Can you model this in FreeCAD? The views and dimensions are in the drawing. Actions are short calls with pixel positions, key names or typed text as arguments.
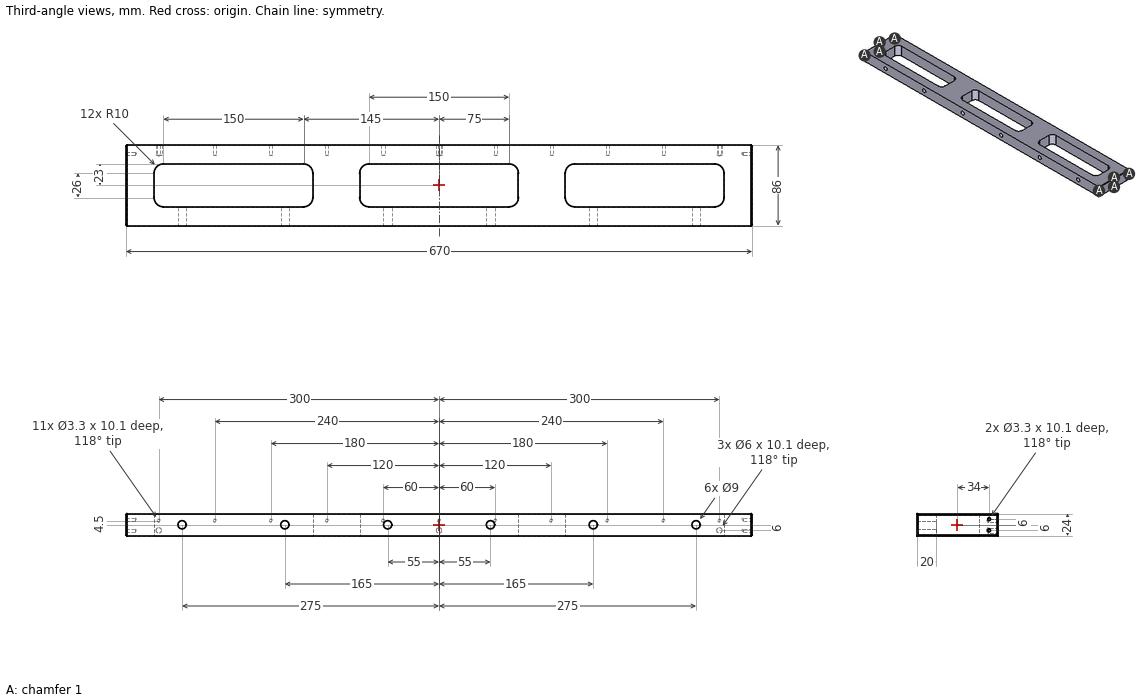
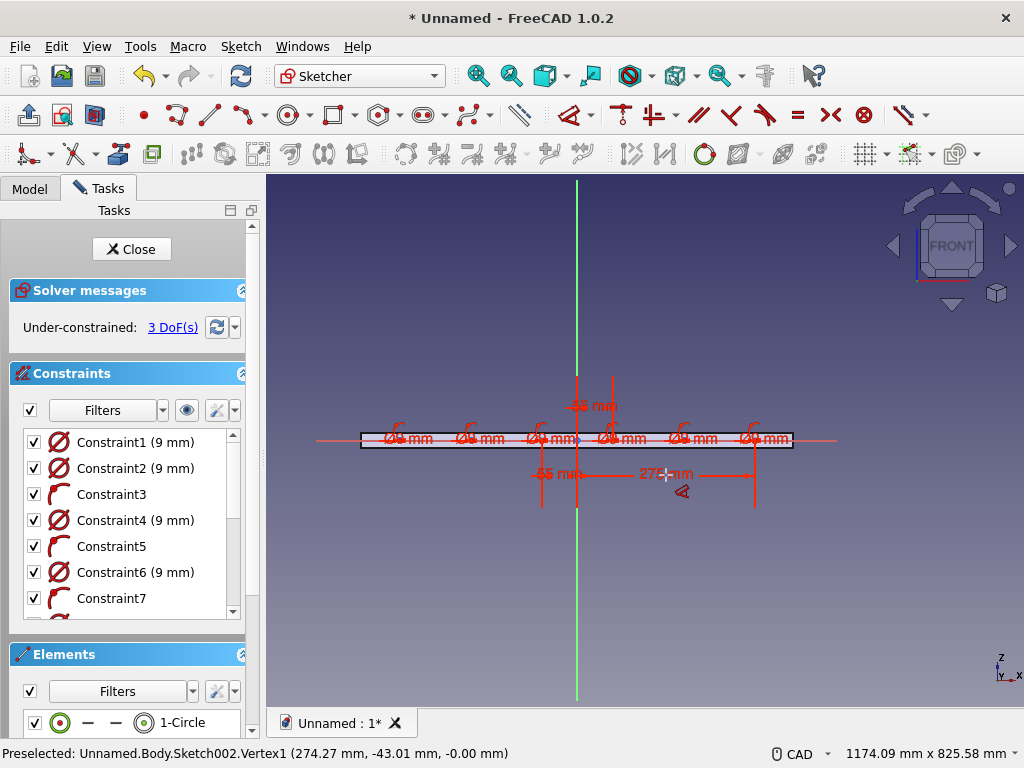
click(399, 441)
click(488, 475)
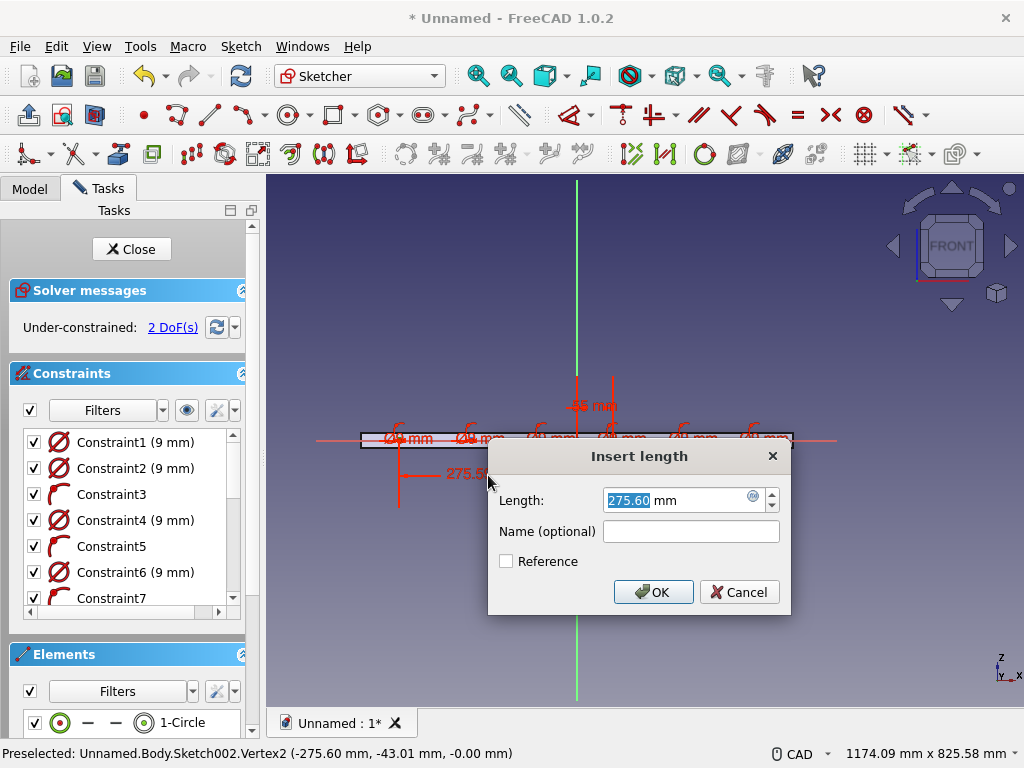
text(275)
key(Return)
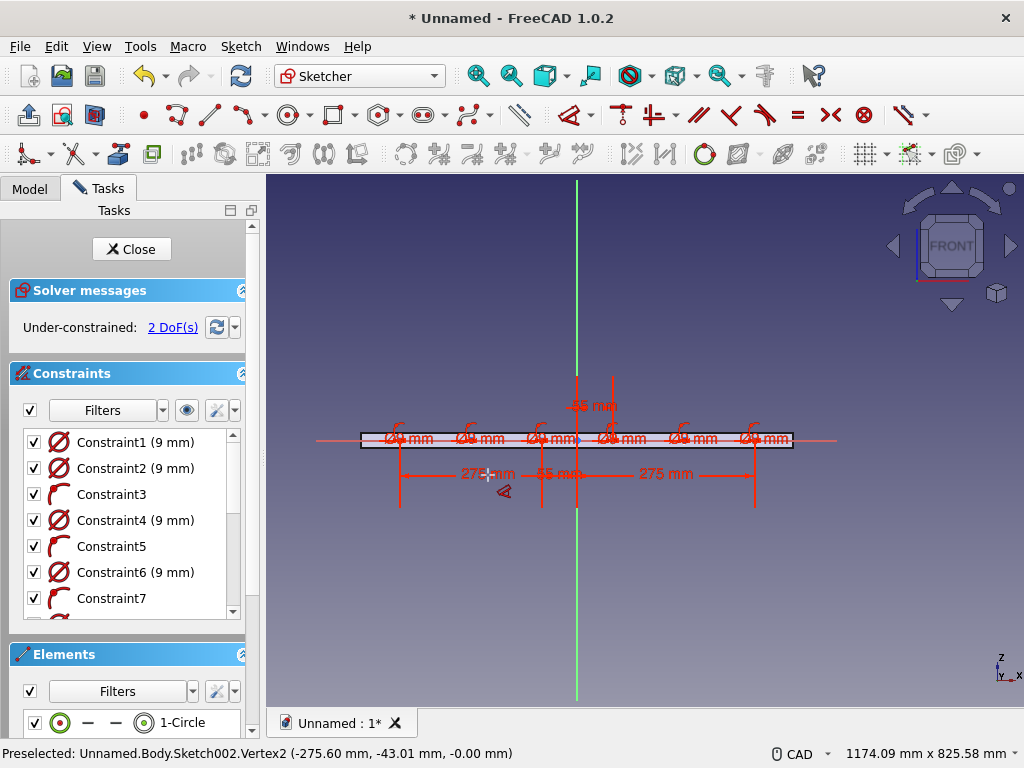
click(471, 441)
click(524, 407)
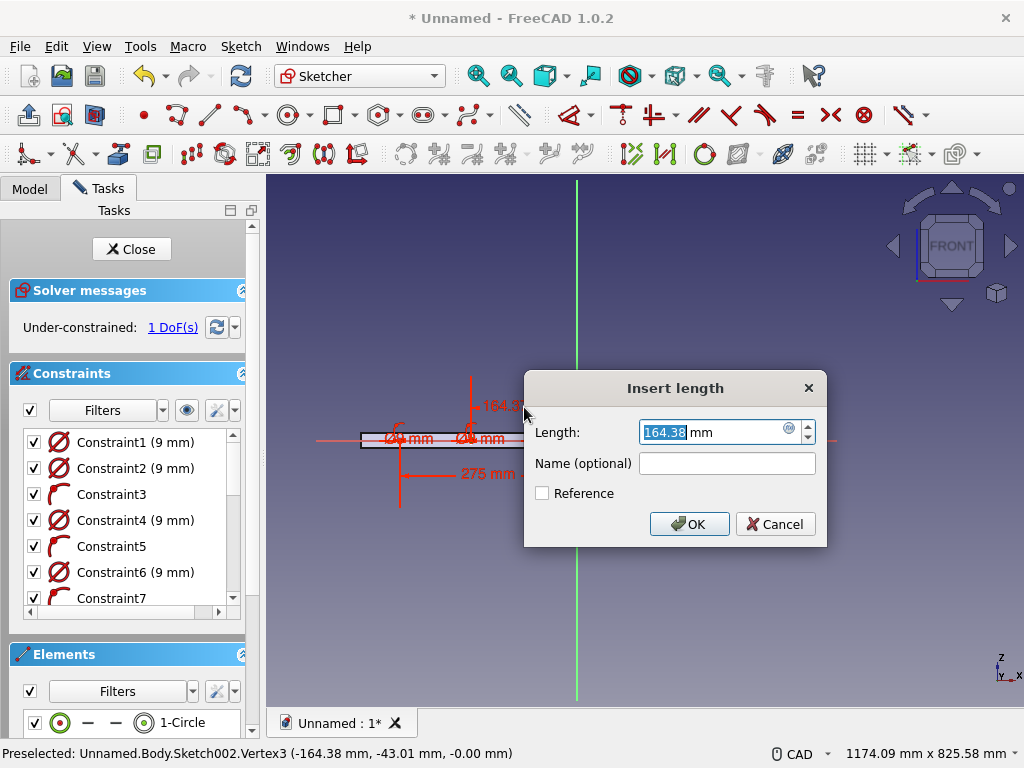
text(165)
key(Return)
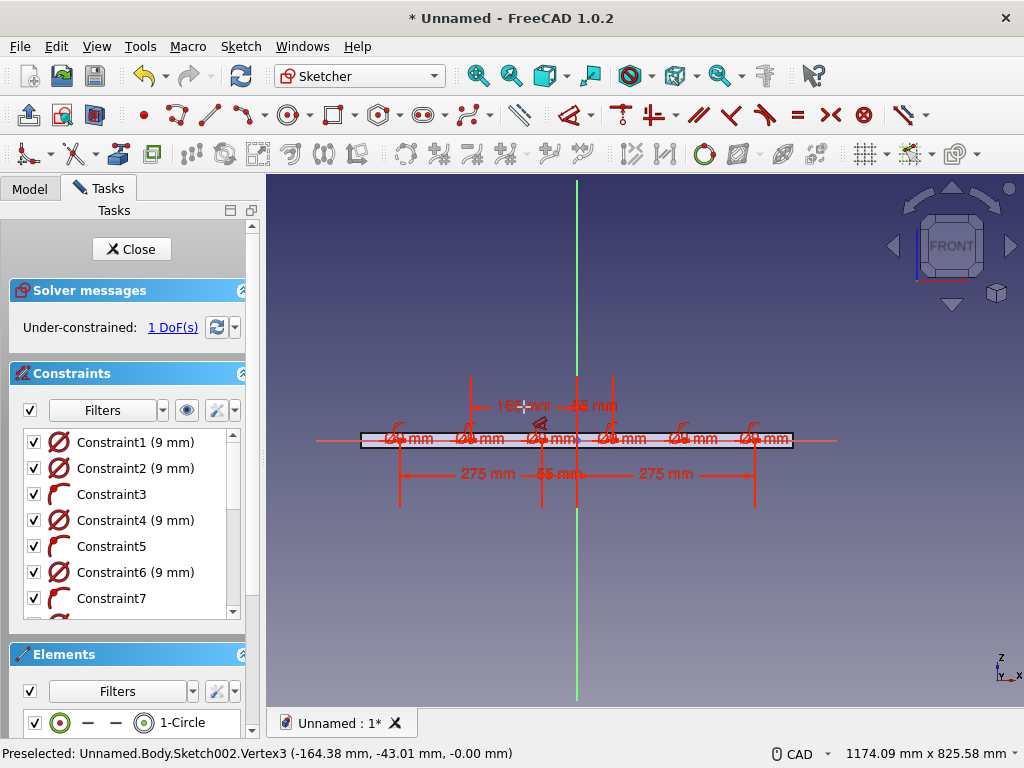
click(684, 441)
click(668, 407)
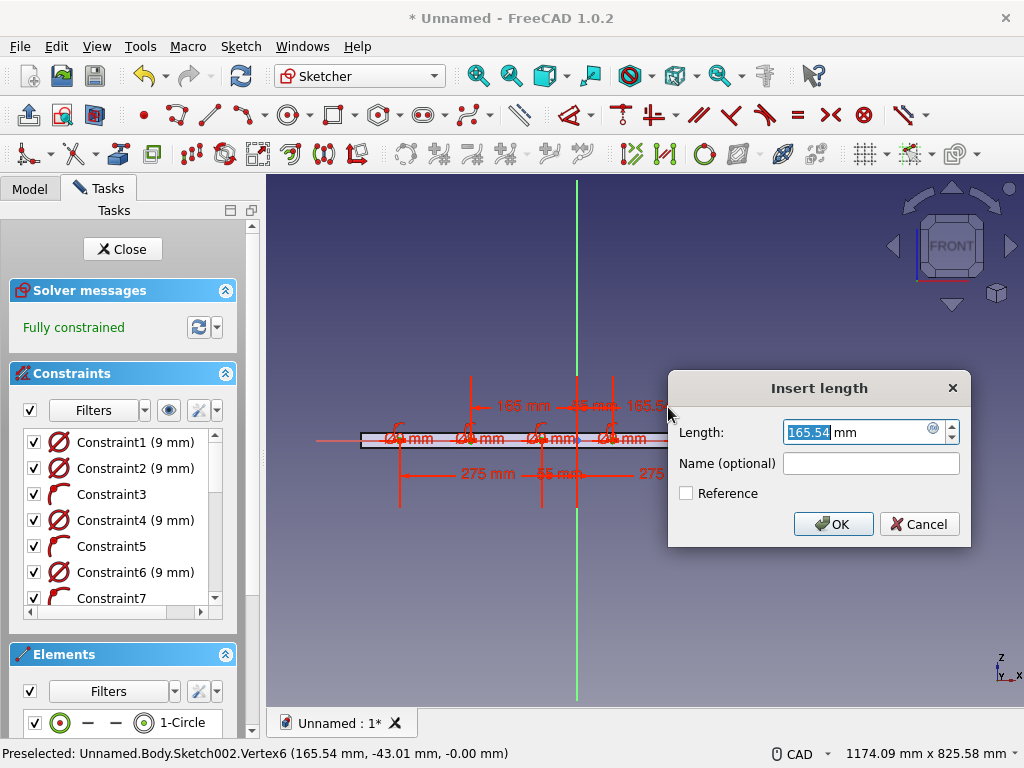
text(165)
key(Return)
key(Escape)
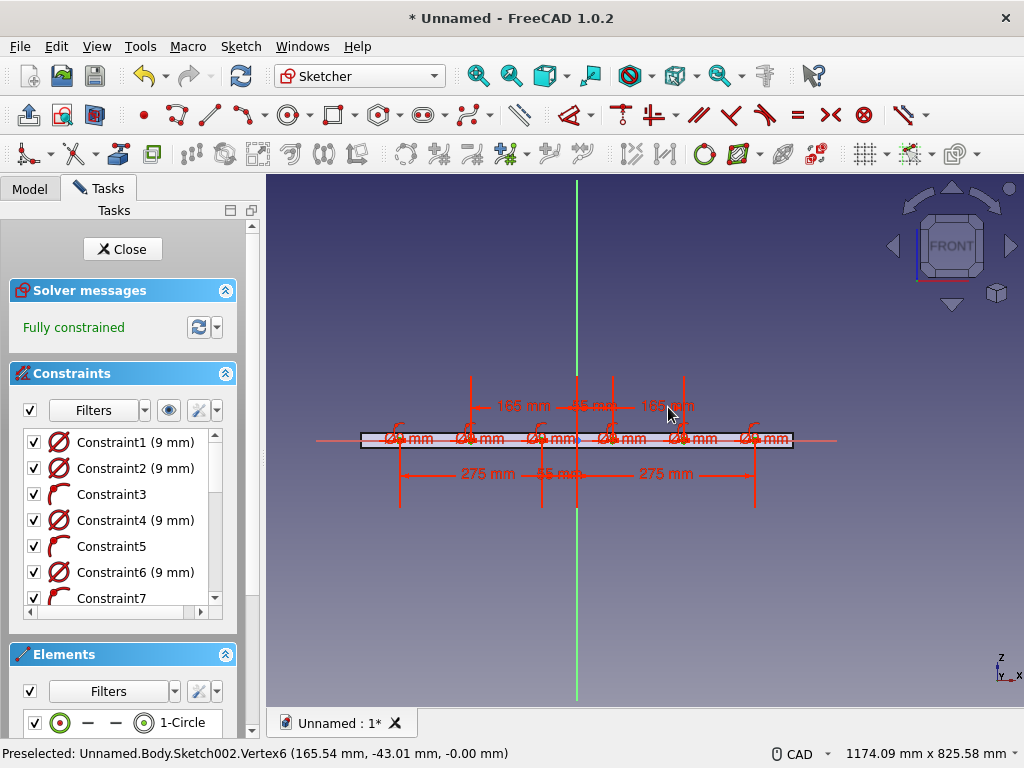
click(123, 249)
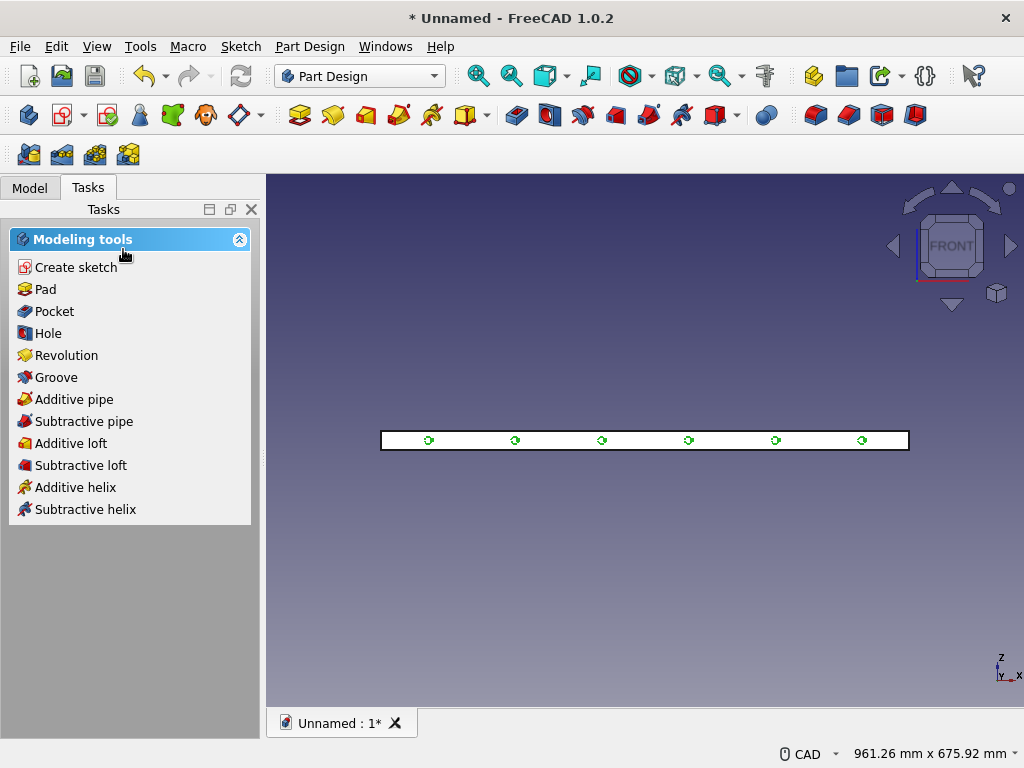
click(517, 116)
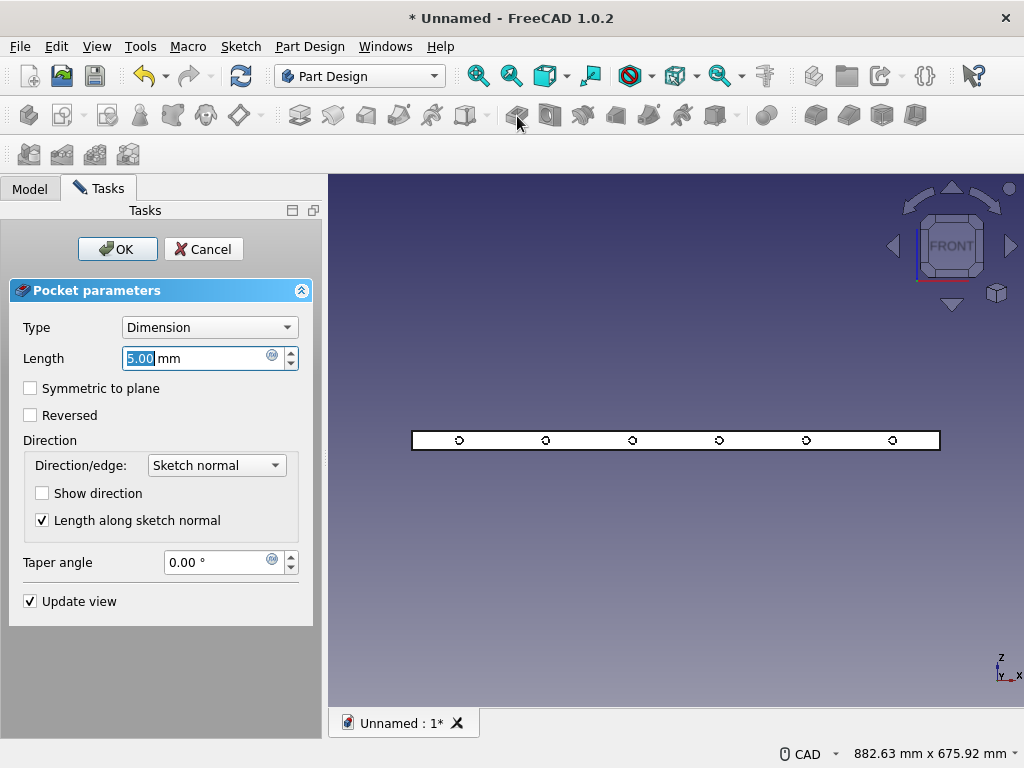
text(20)
key(Tab)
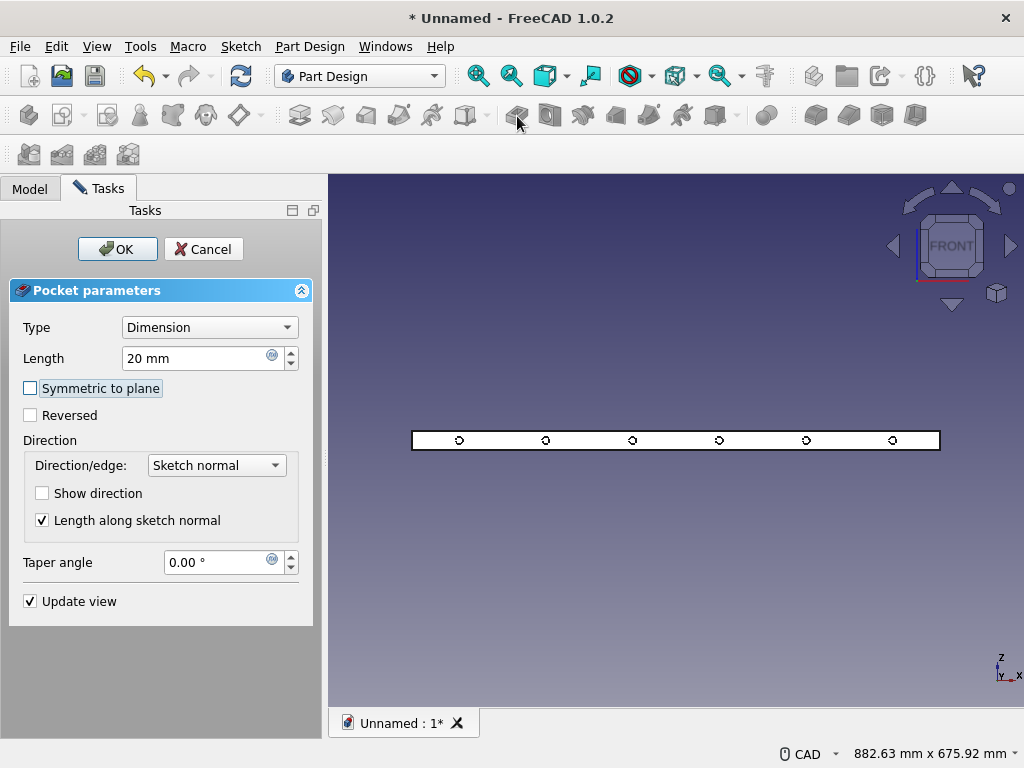
click(118, 249)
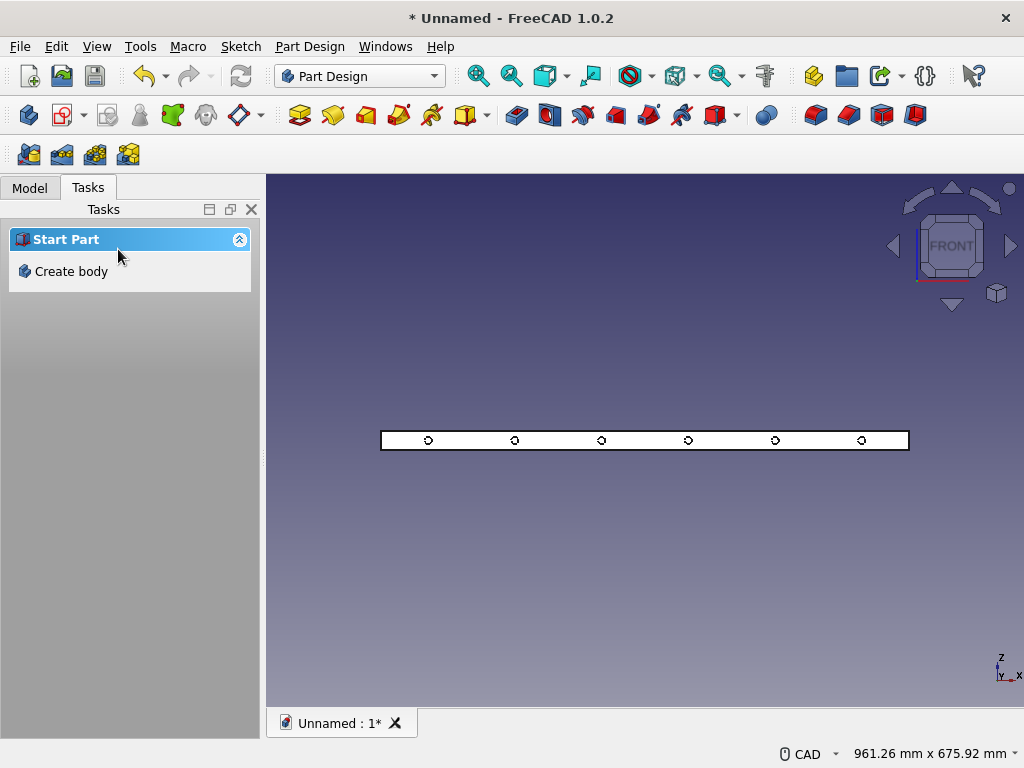
key(4)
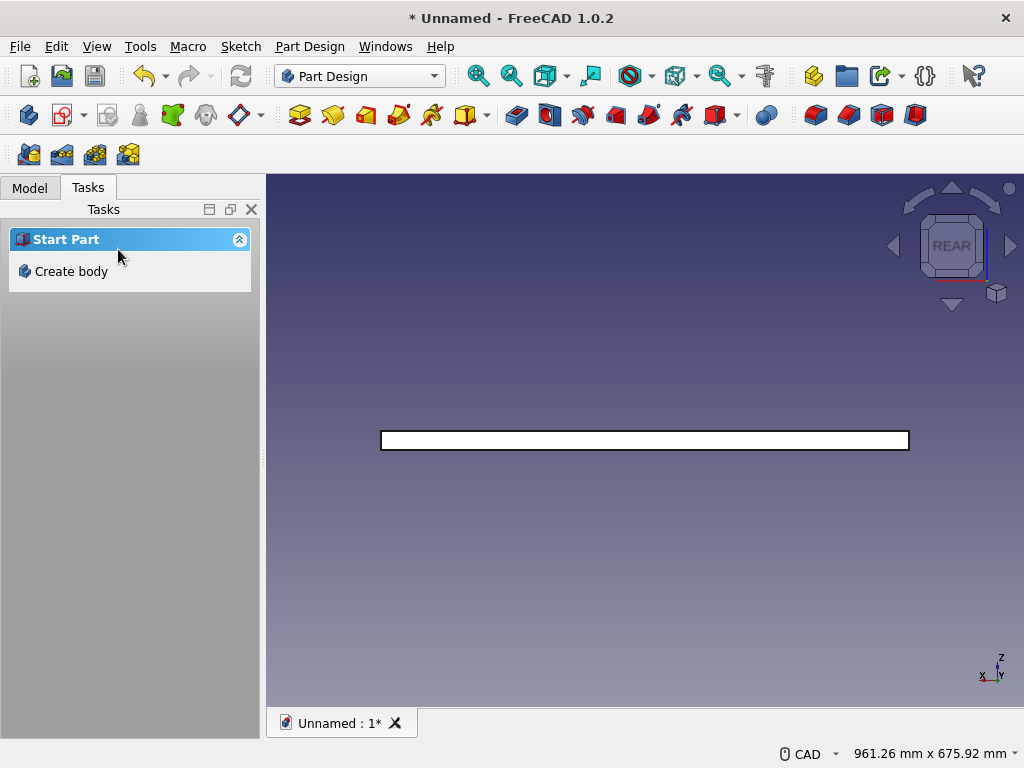
click(419, 439)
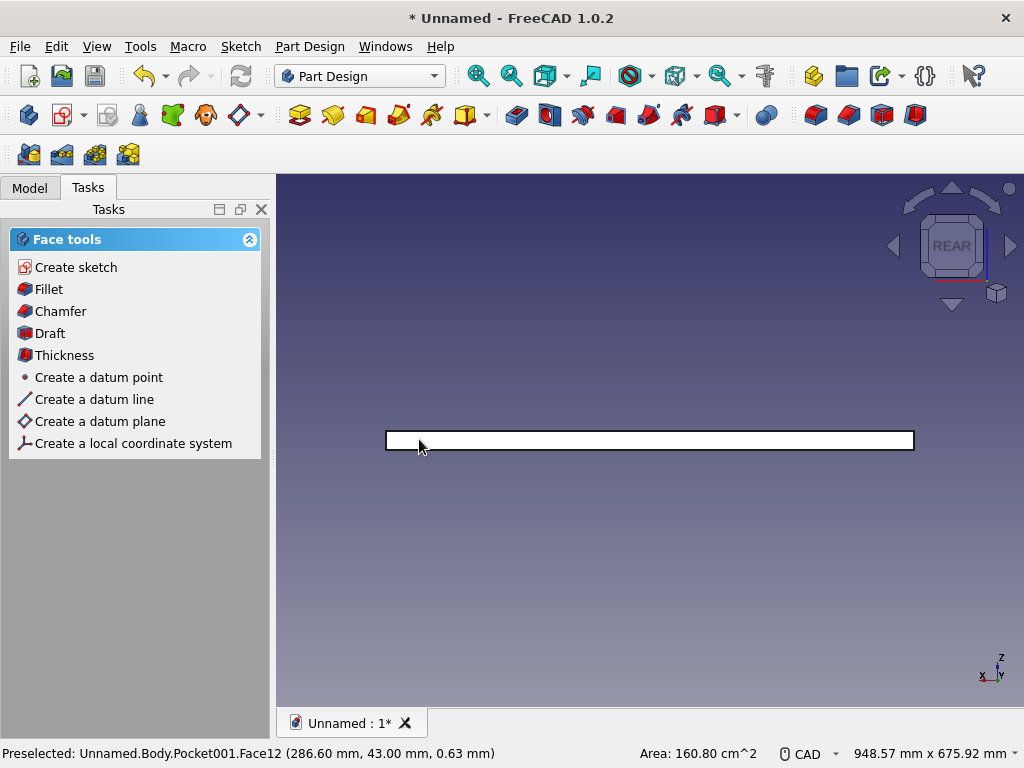
click(62, 116)